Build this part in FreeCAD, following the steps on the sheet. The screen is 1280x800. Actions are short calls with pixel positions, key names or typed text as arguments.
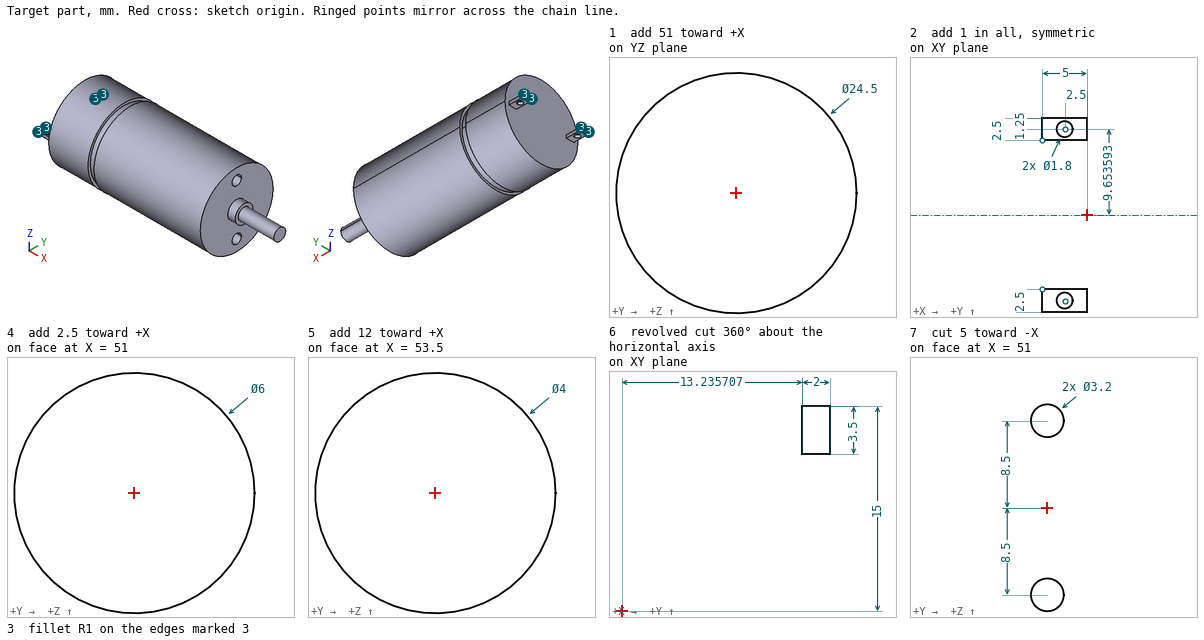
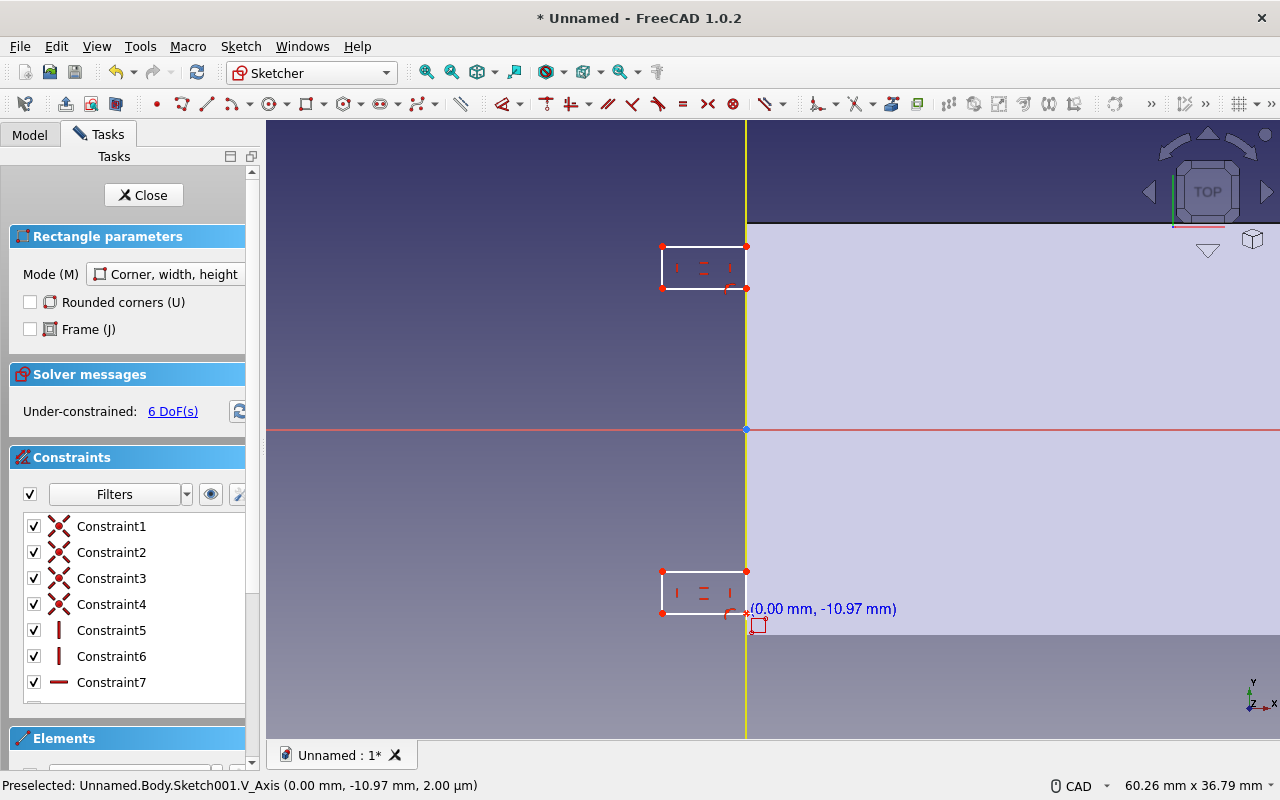
click(268, 104)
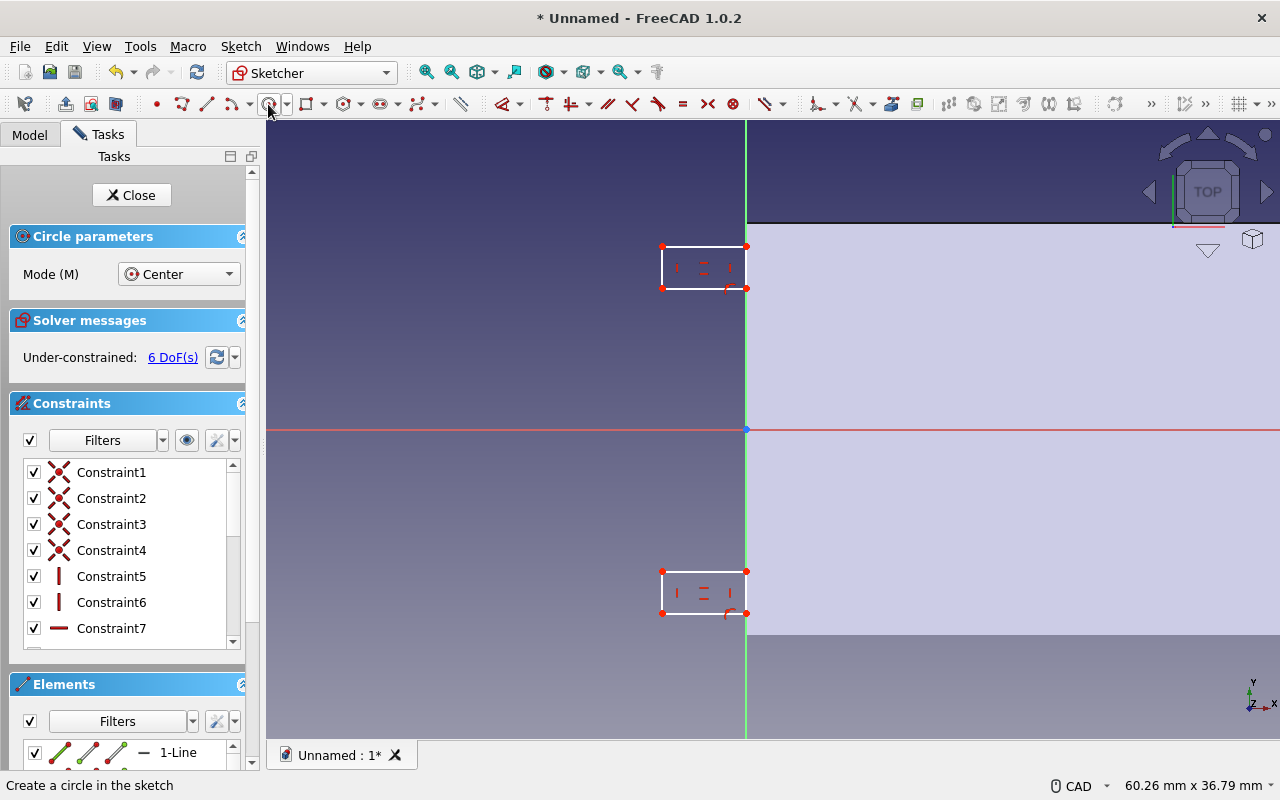
scroll(704, 267, up, 3)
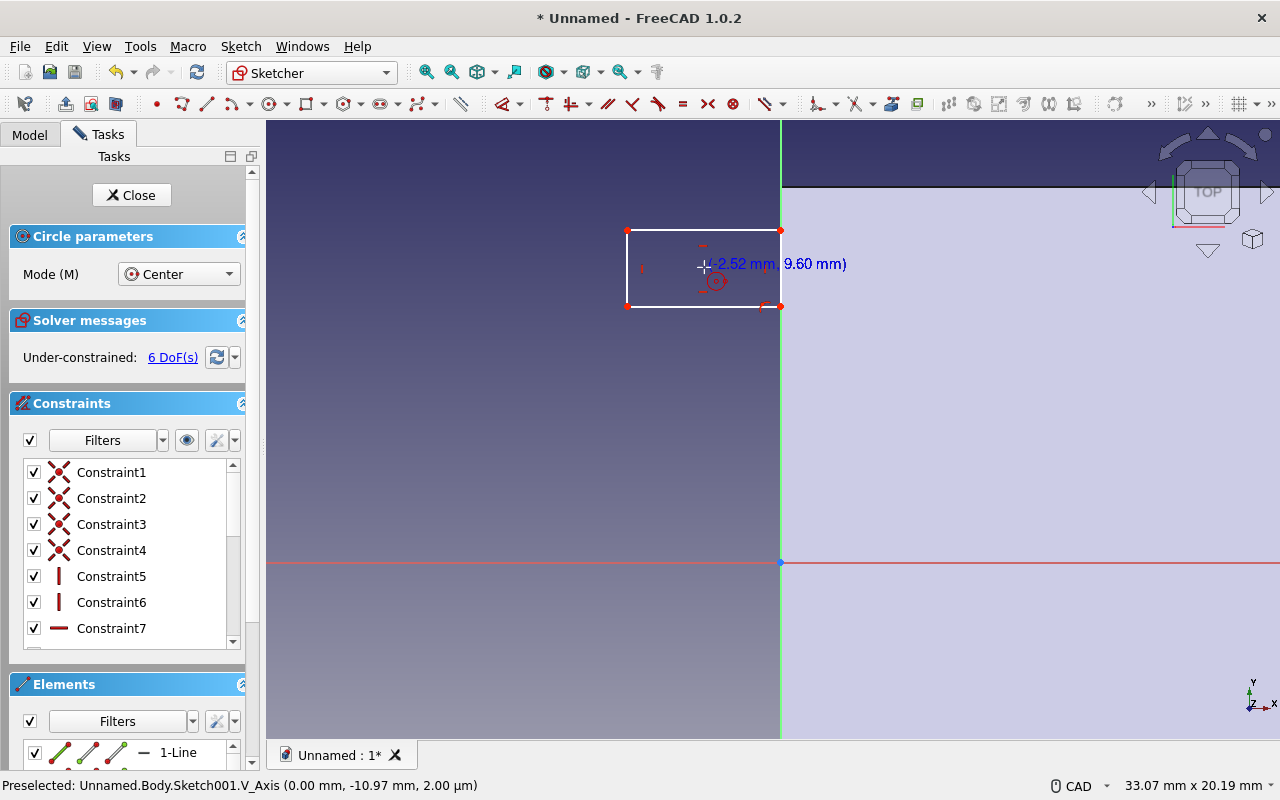
click(704, 267)
move(724, 247)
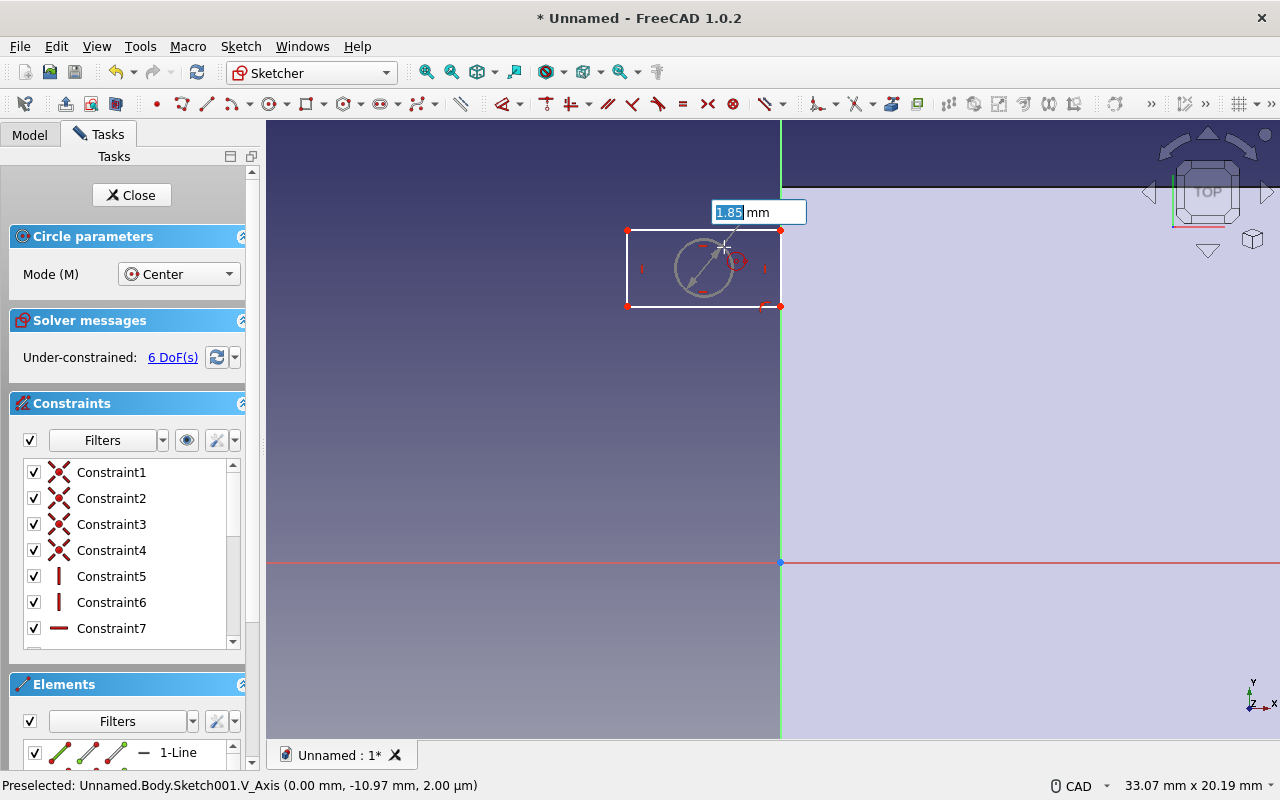
text(1.8)
key(Return)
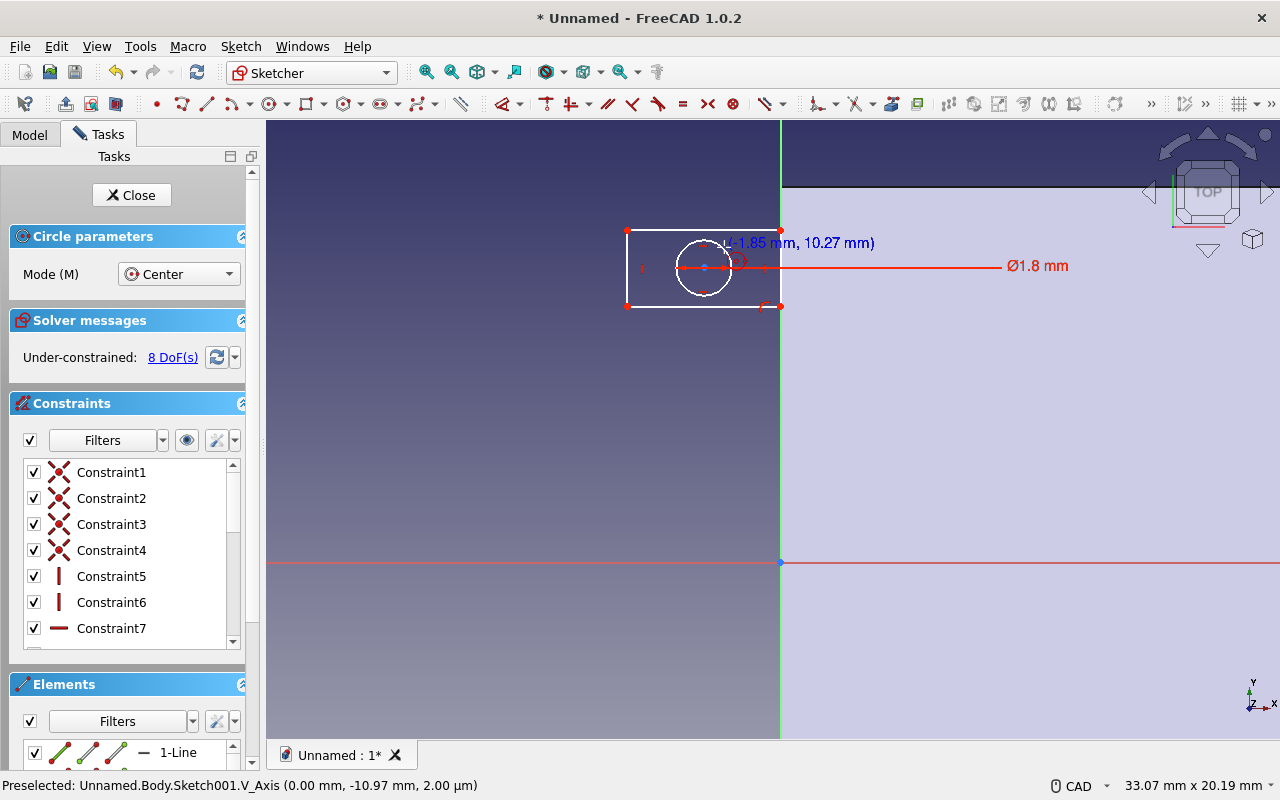
scroll(705, 267, down, 3)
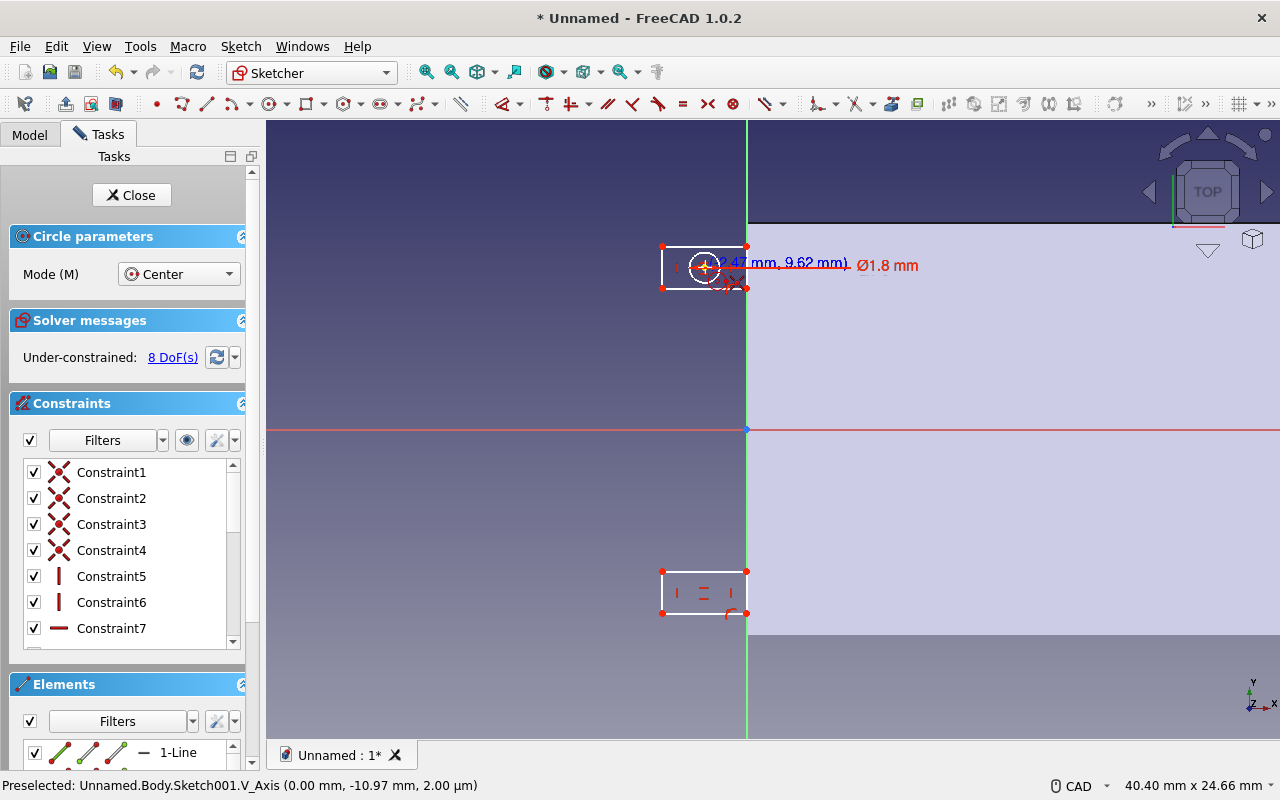
scroll(705, 592, up, 3)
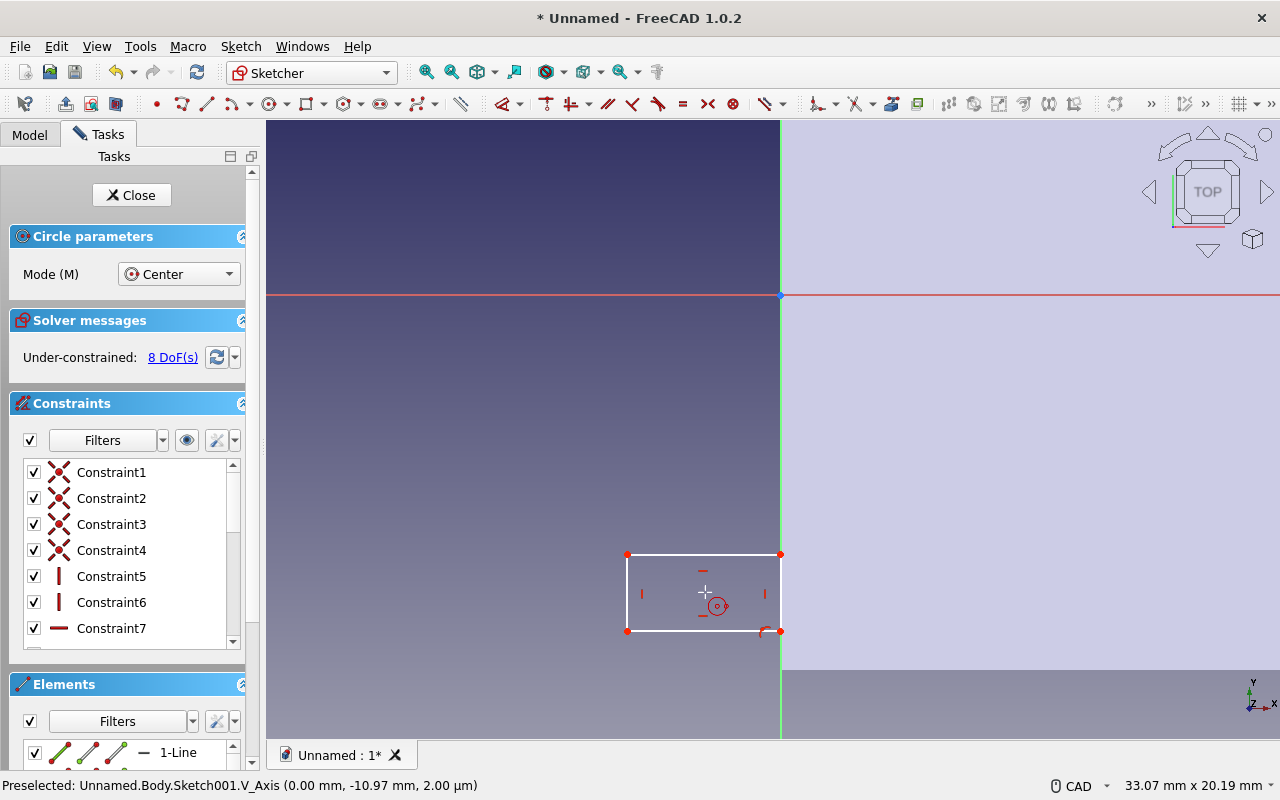
click(704, 591)
move(724, 572)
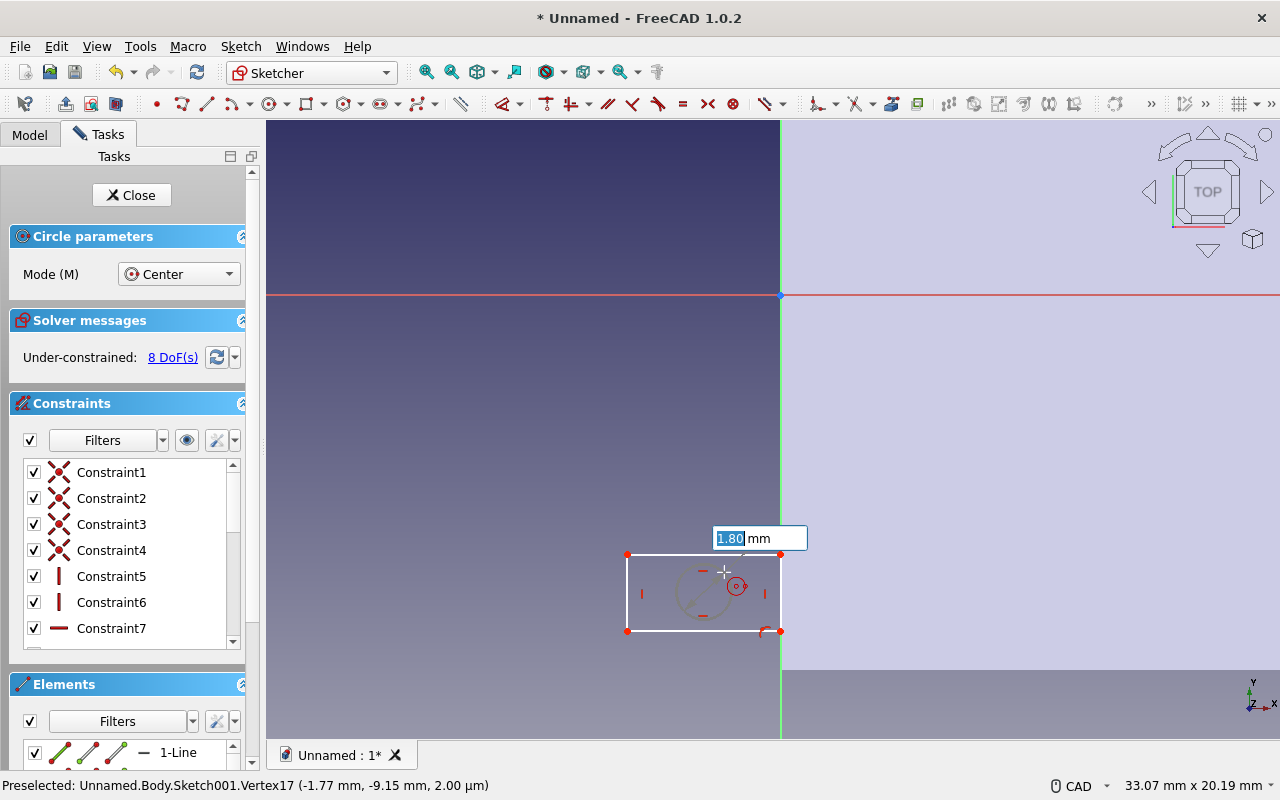
text(1.8)
key(Return)
key(Escape)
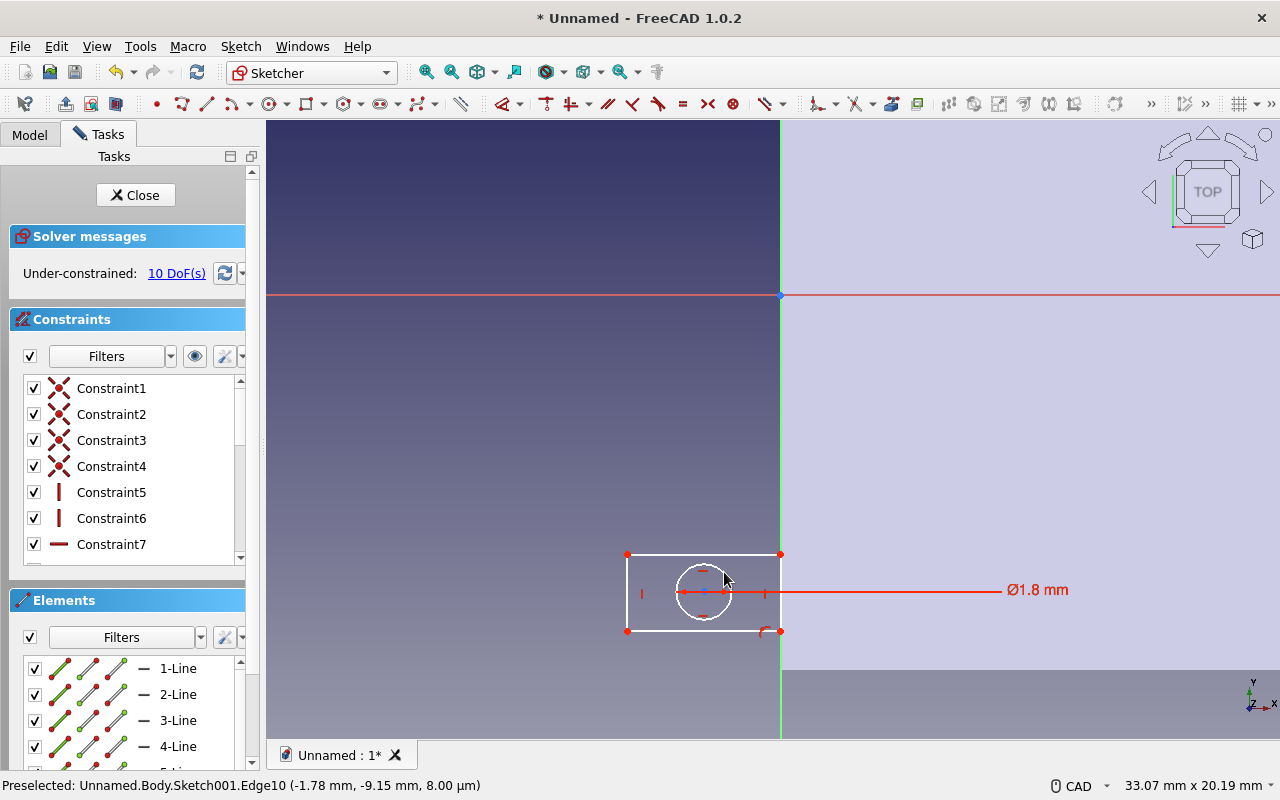
scroll(705, 593, down, 3)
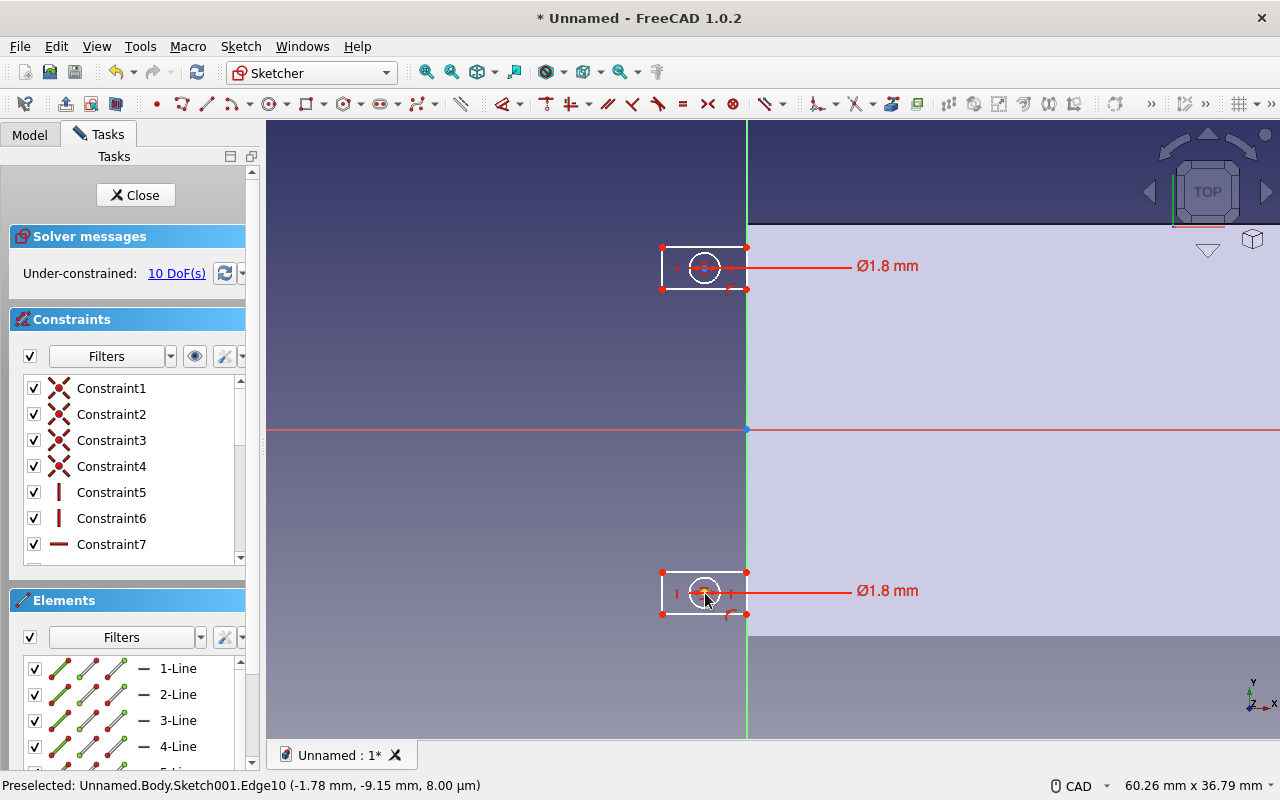
click(705, 268)